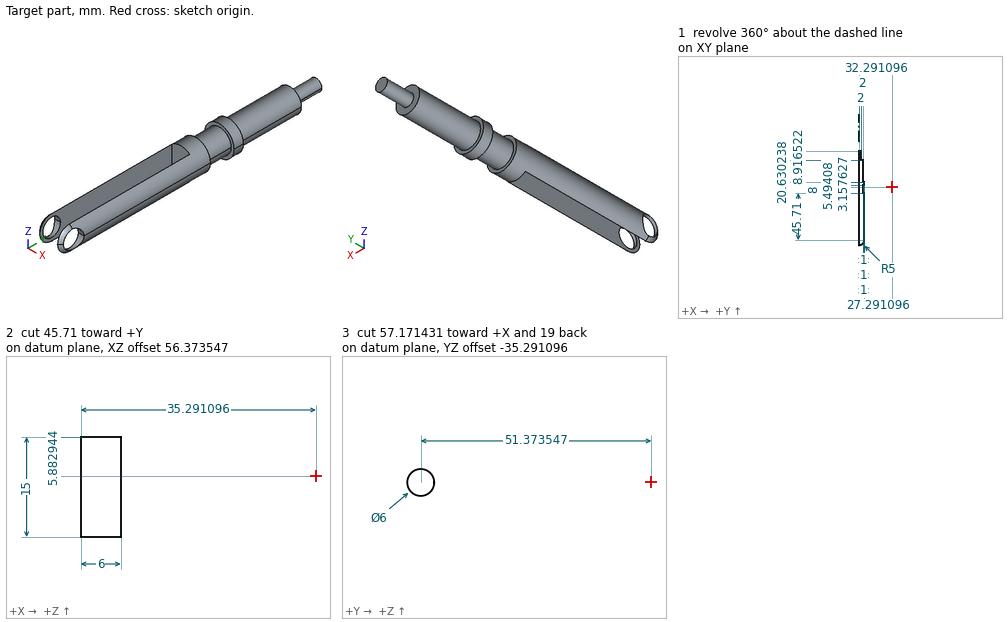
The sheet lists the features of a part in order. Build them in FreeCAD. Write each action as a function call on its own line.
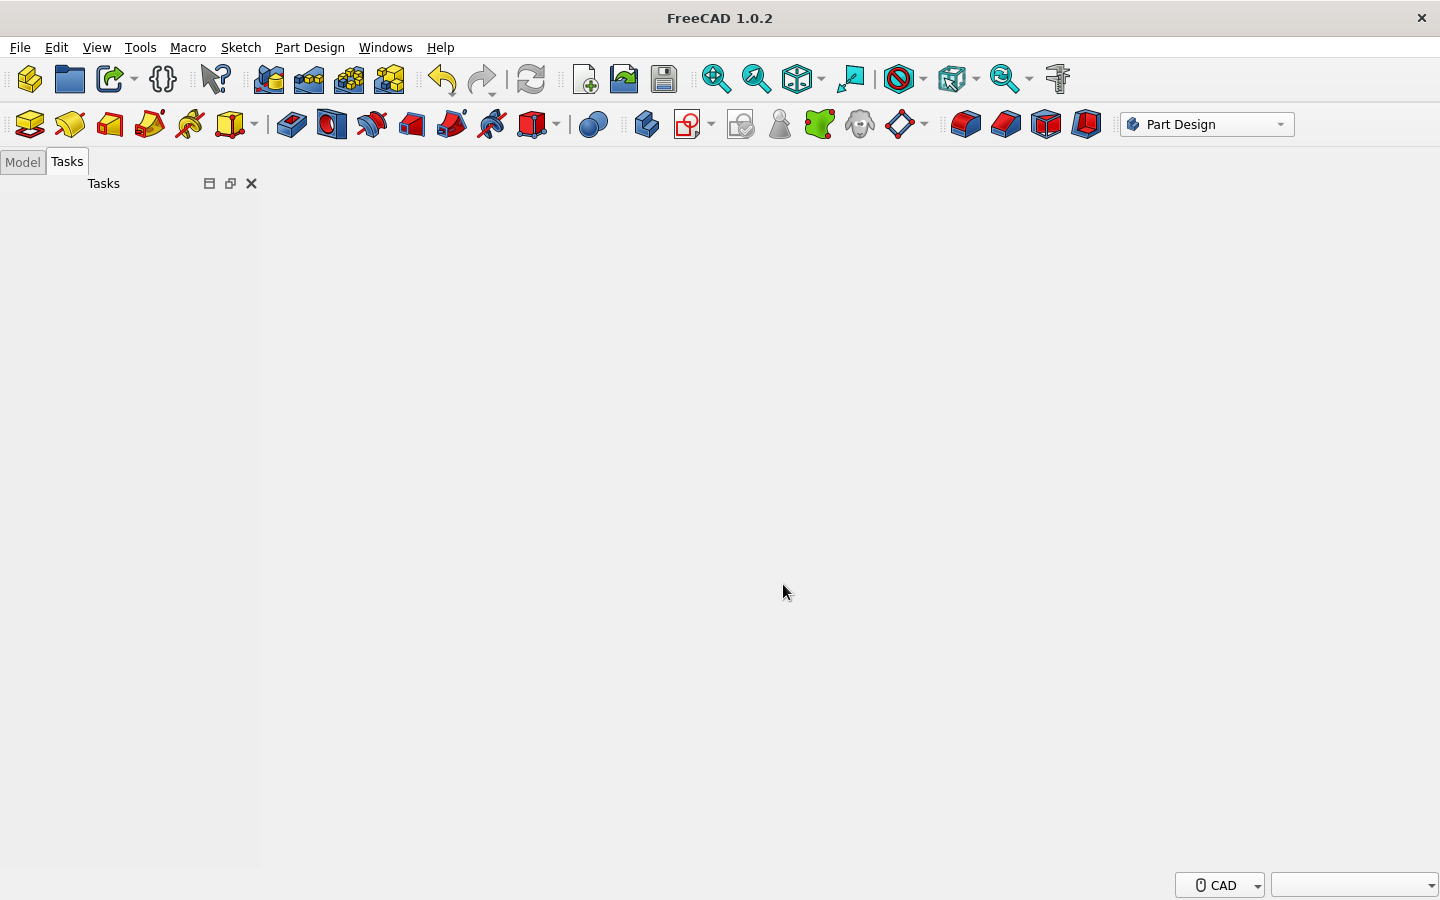
click(584, 80)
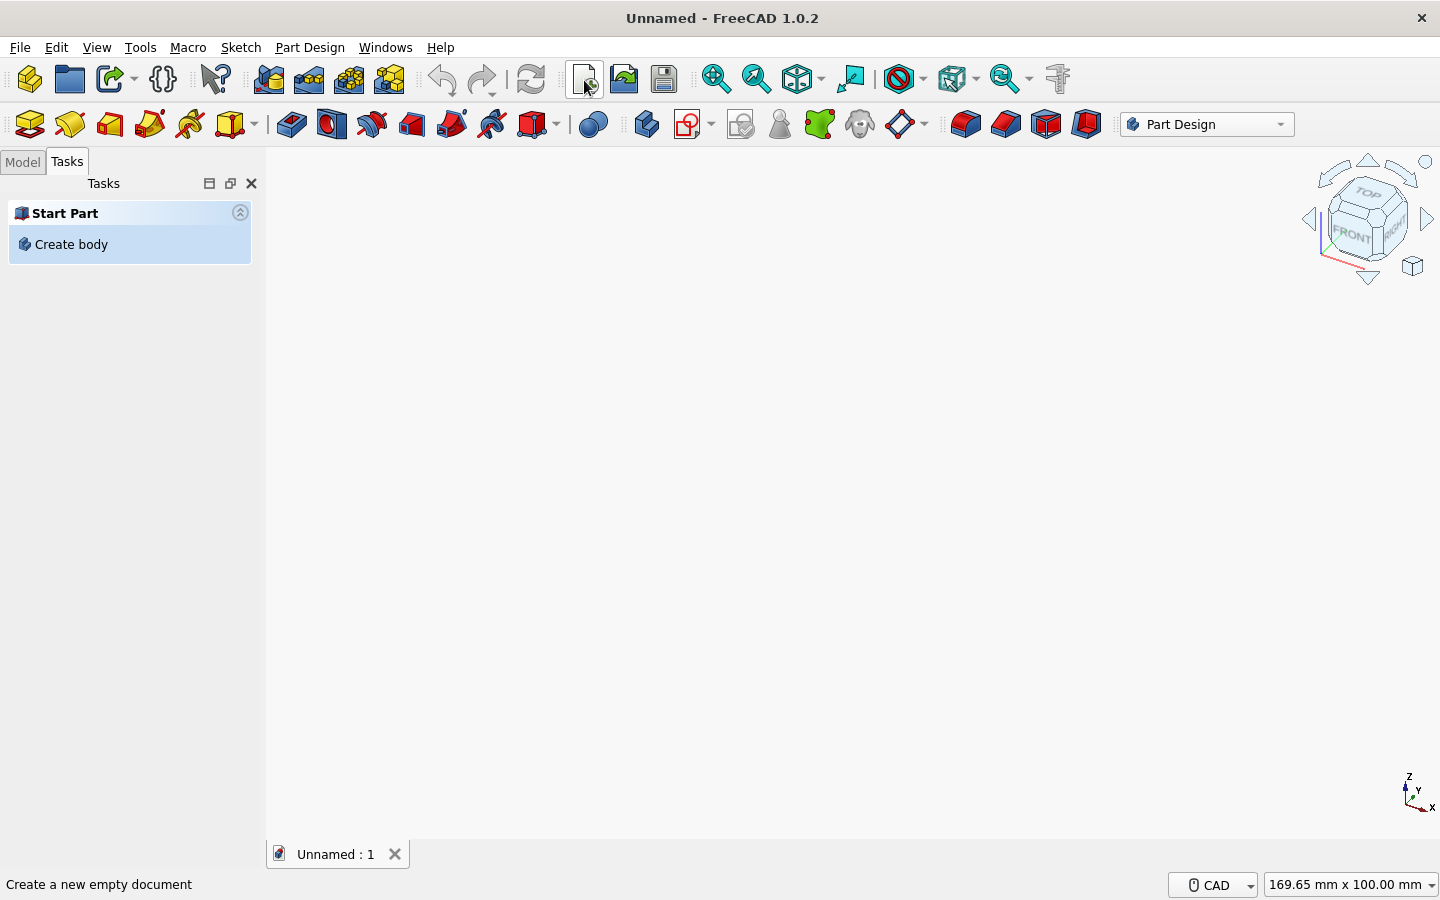
click(688, 124)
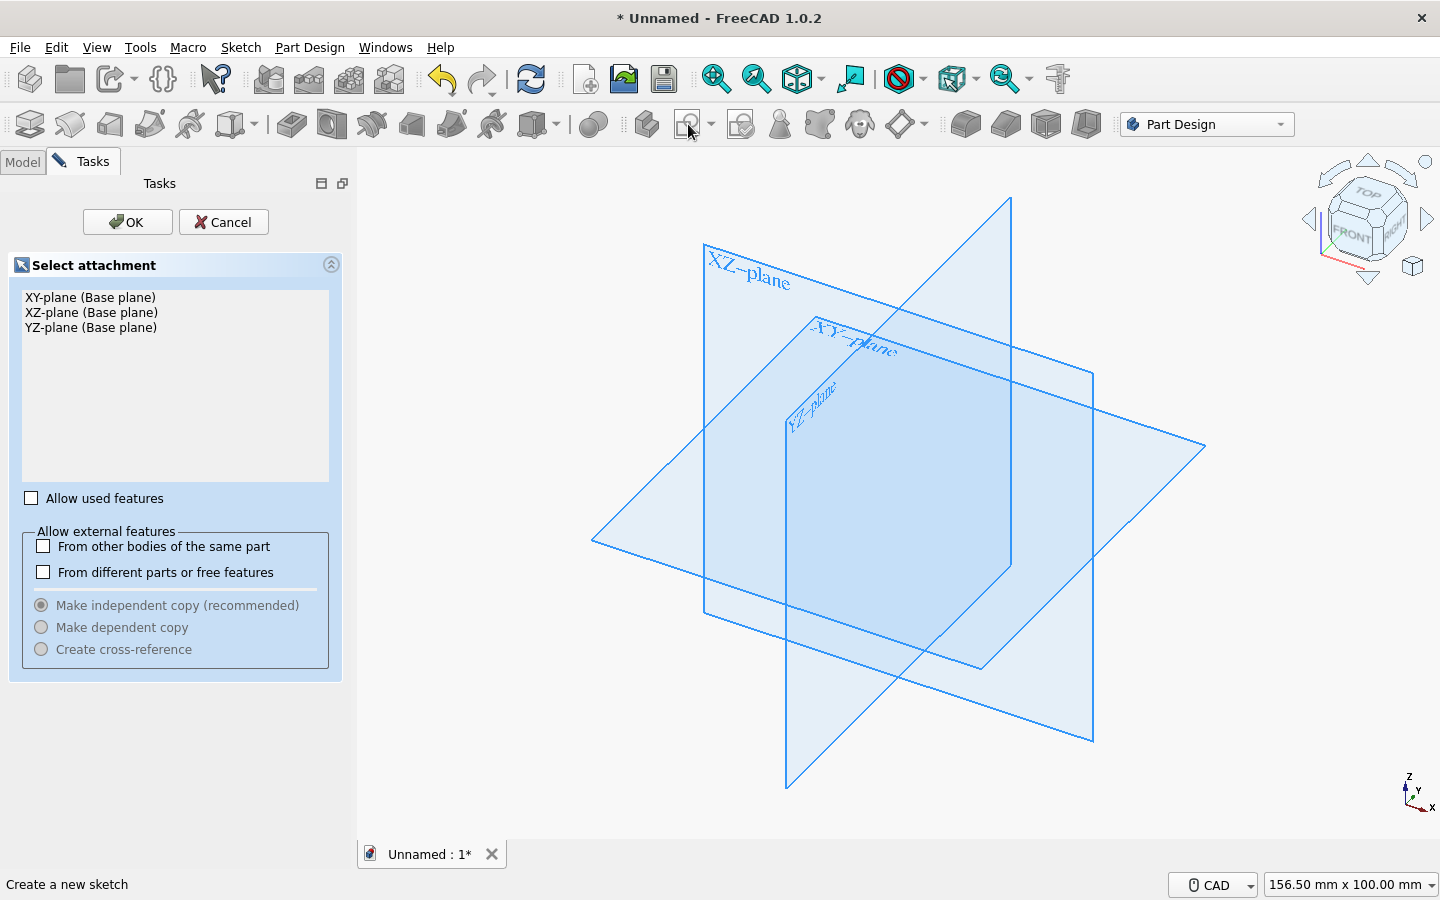
click(82, 298)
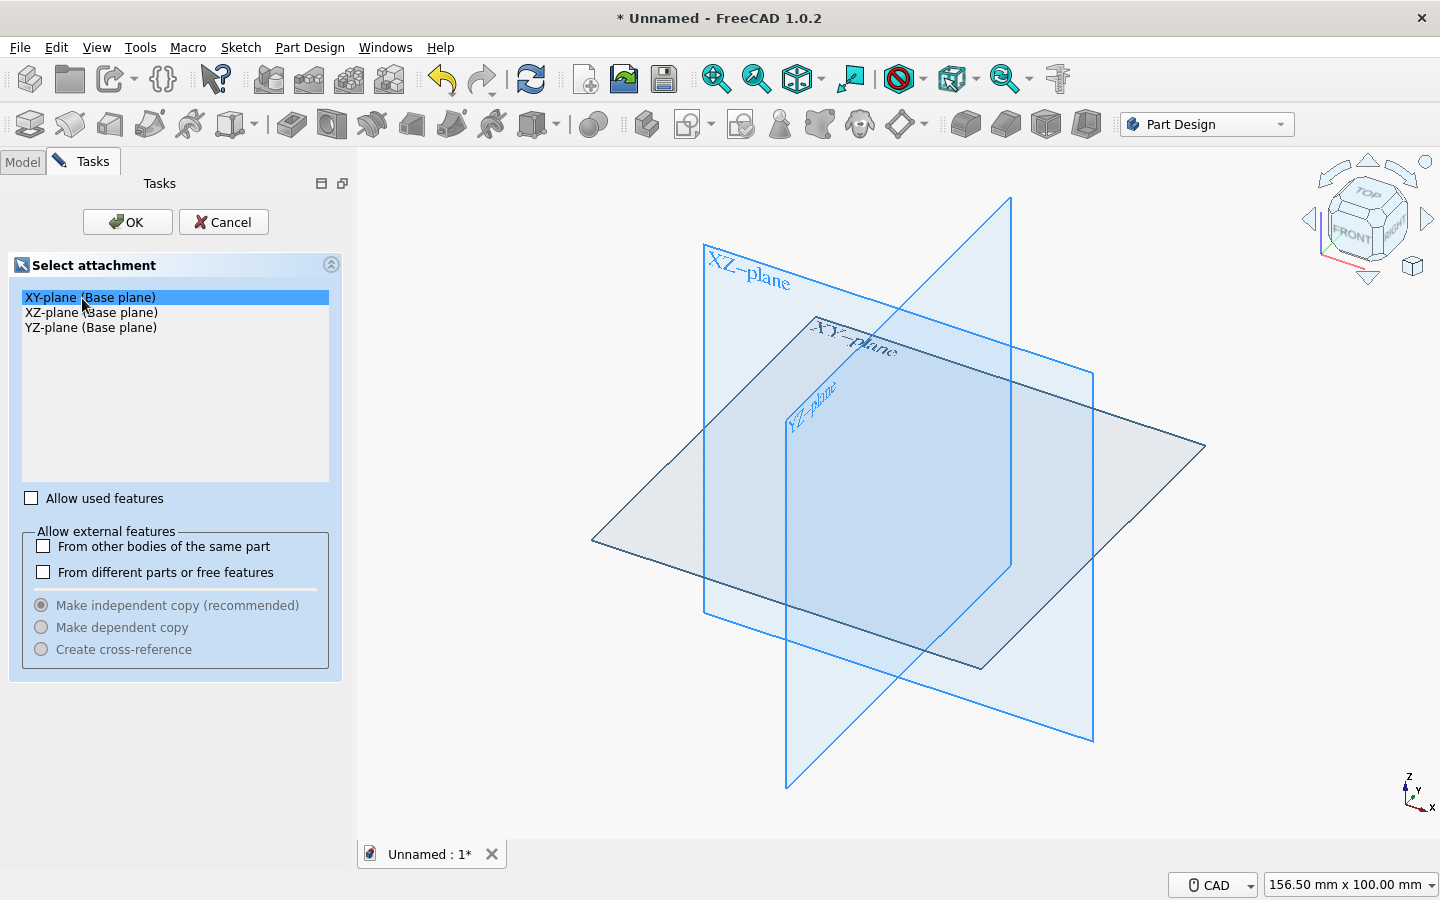
click(128, 222)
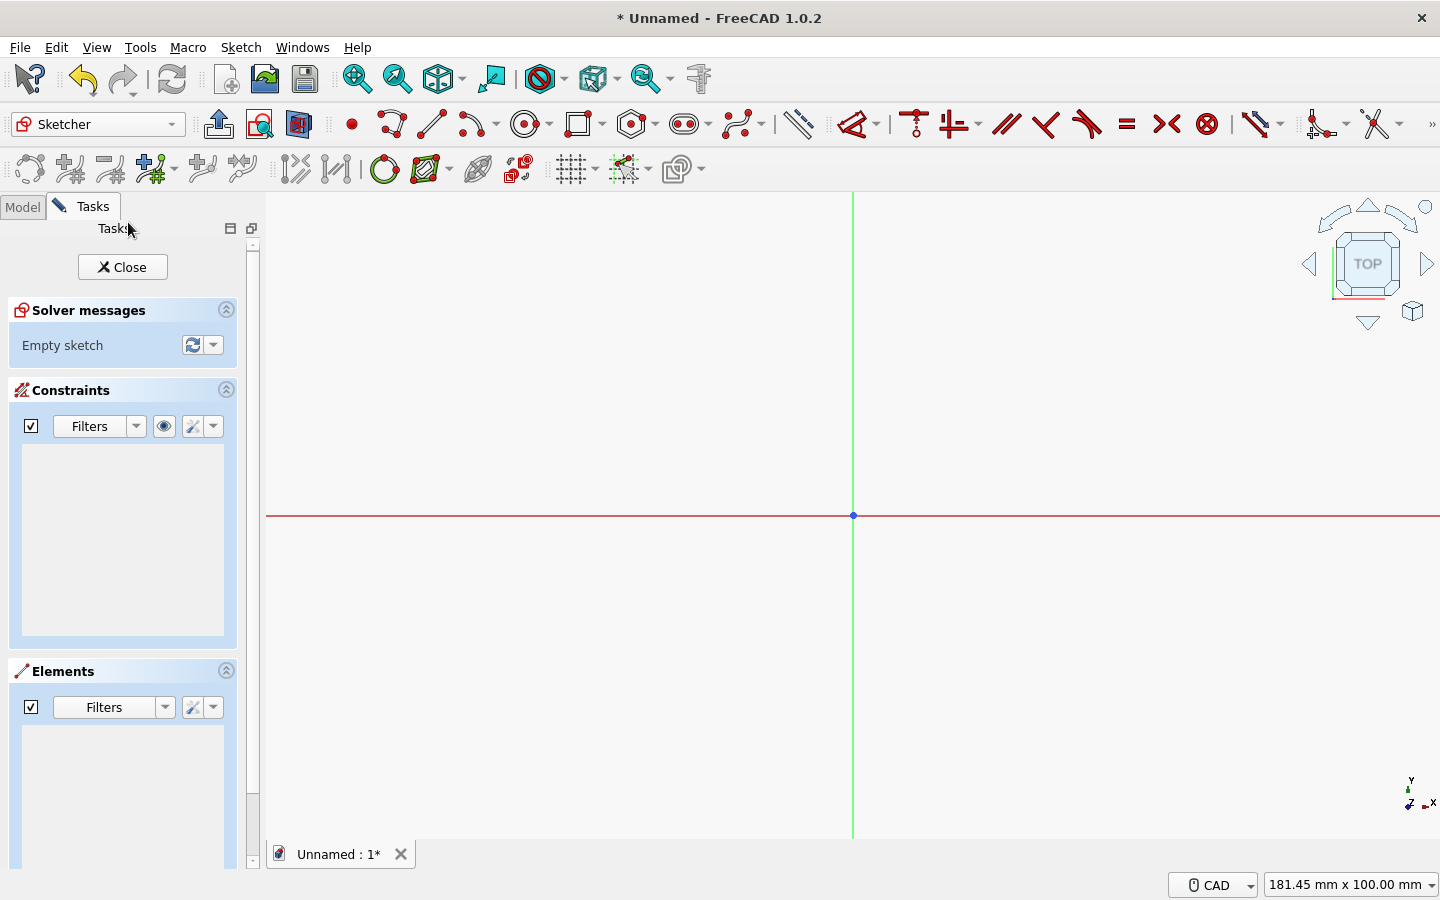
scroll(828, 575, down, 3)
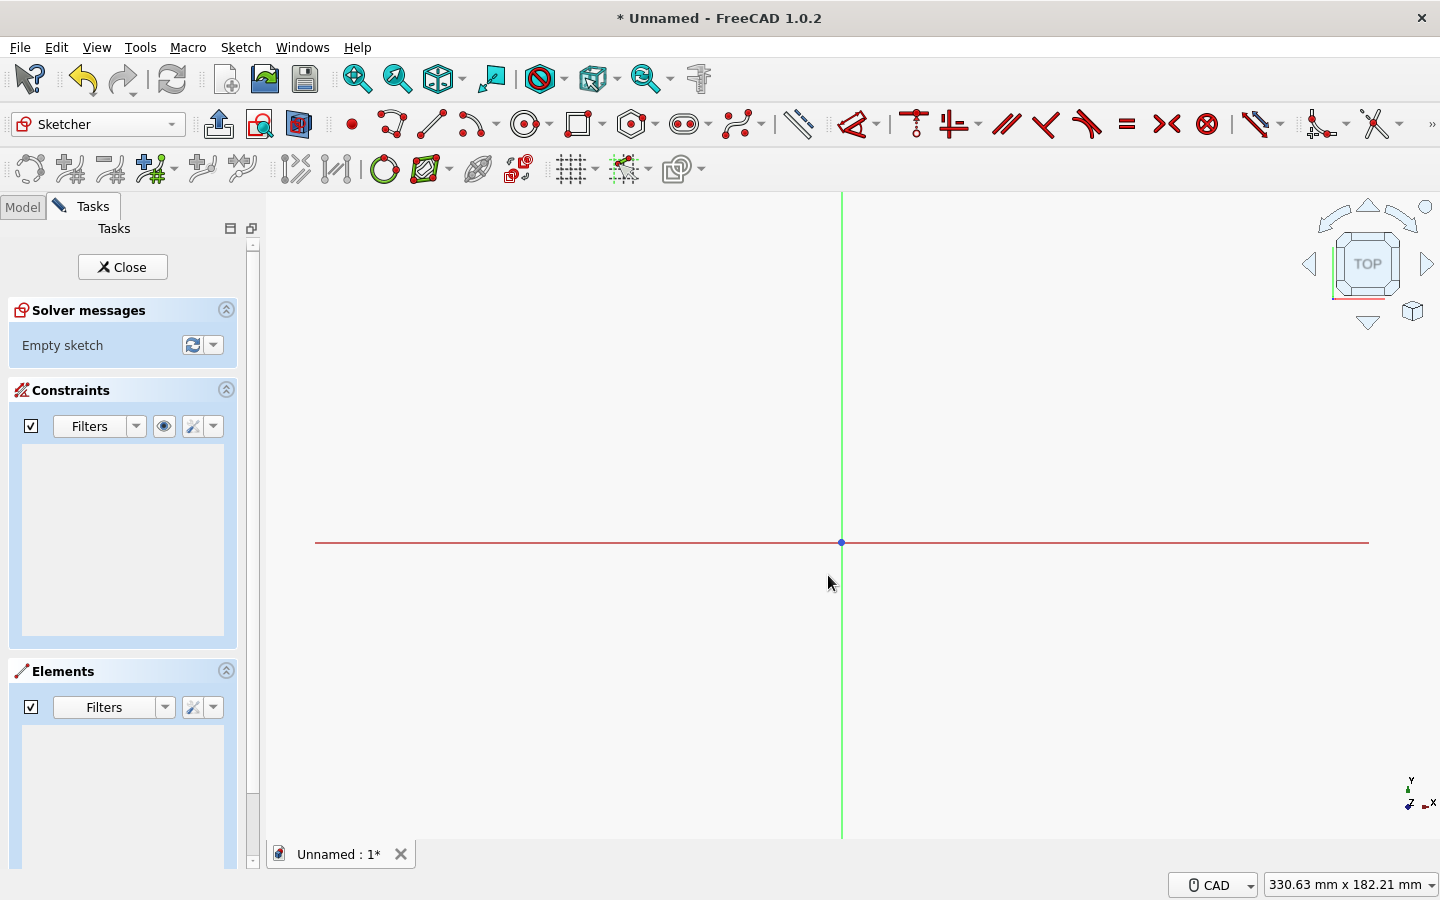
click(392, 124)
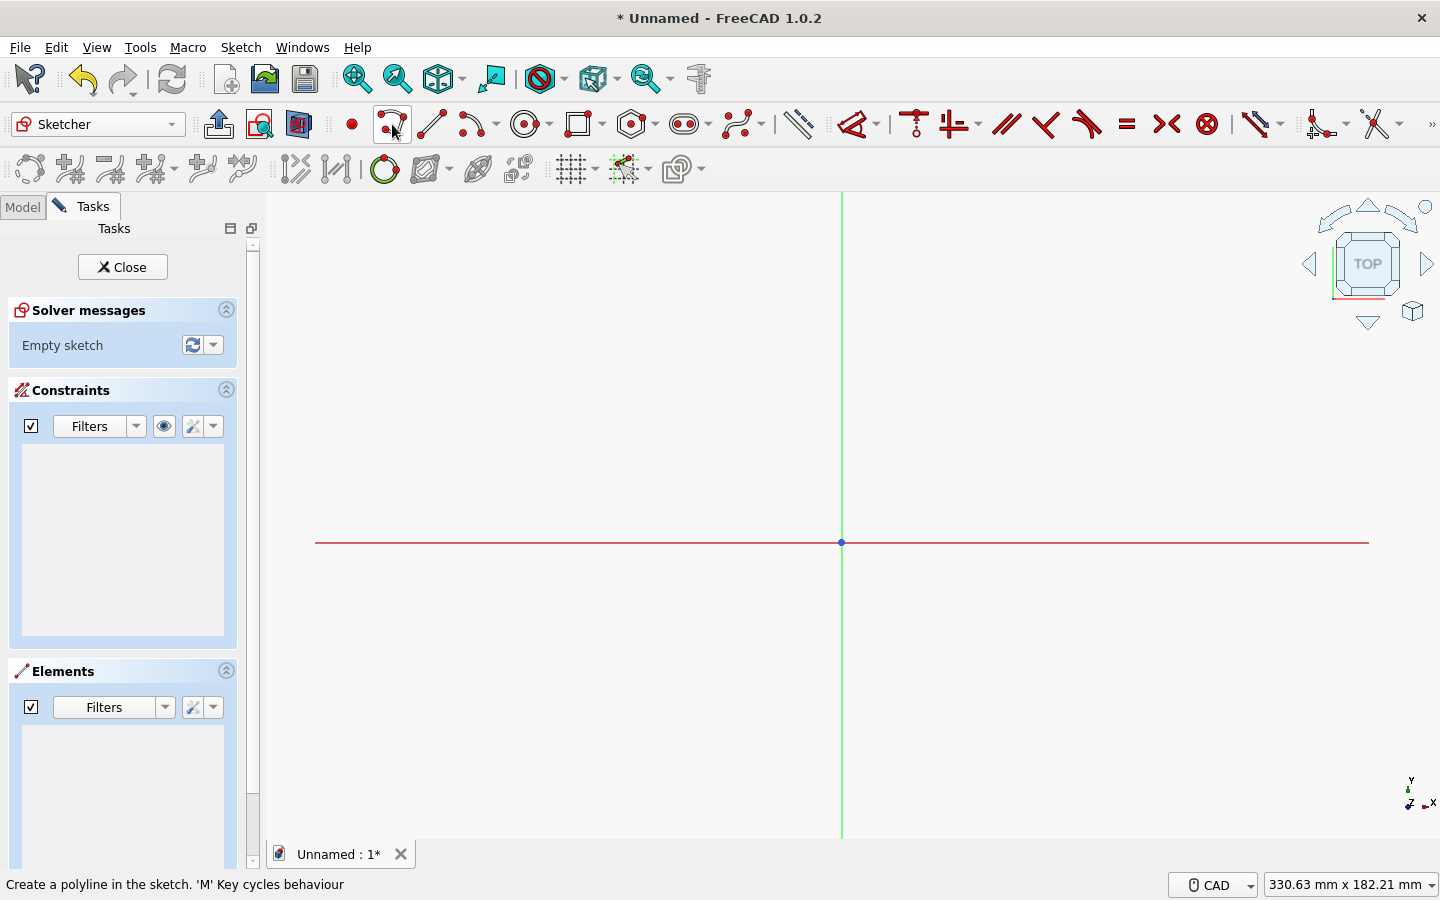
click(745, 725)
click(745, 563)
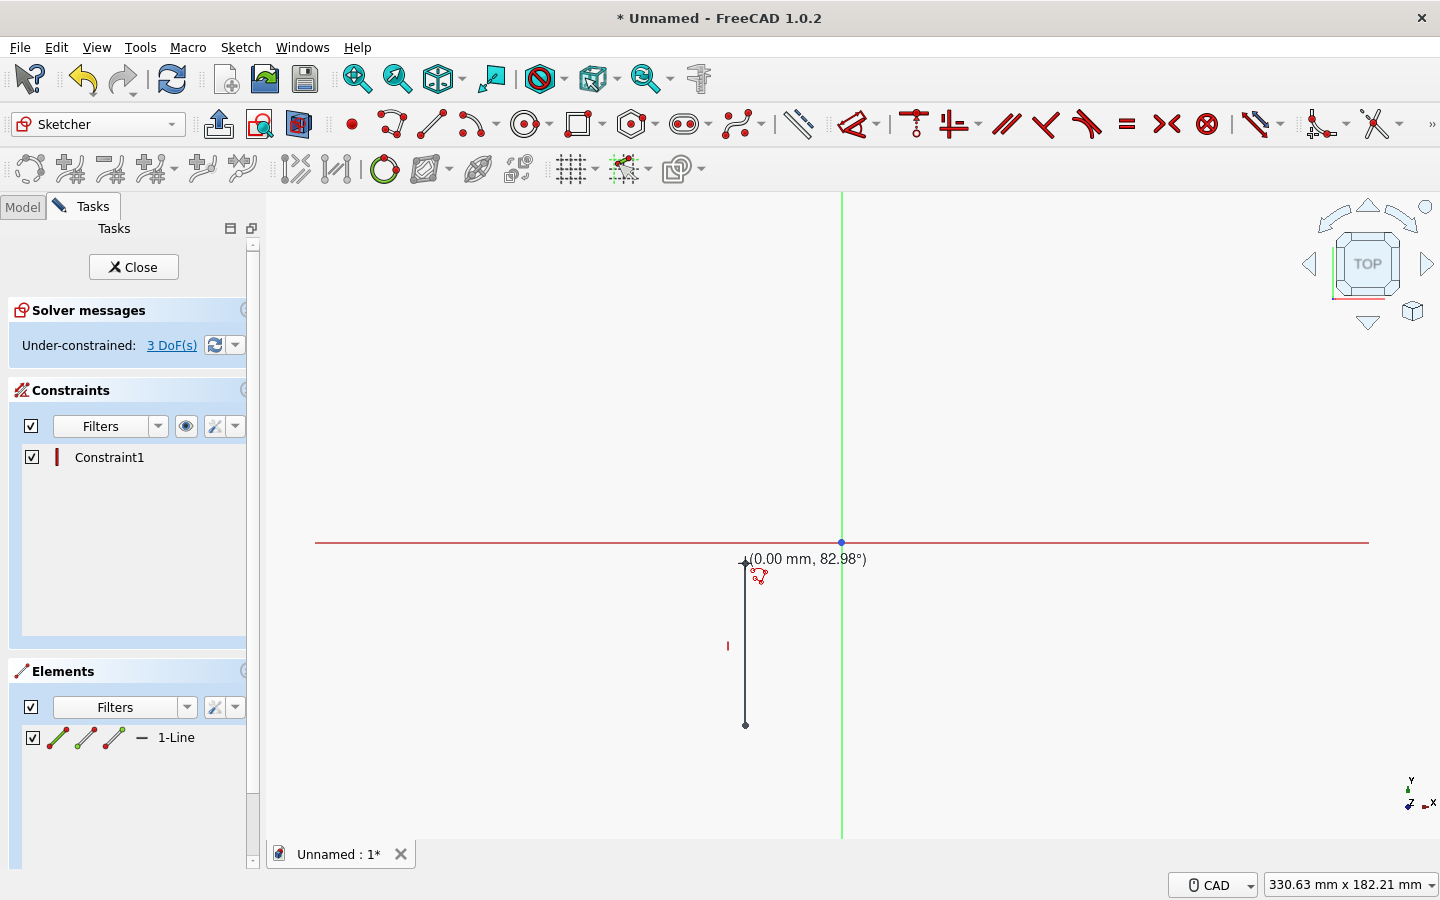
scroll(741, 563, up, 8)